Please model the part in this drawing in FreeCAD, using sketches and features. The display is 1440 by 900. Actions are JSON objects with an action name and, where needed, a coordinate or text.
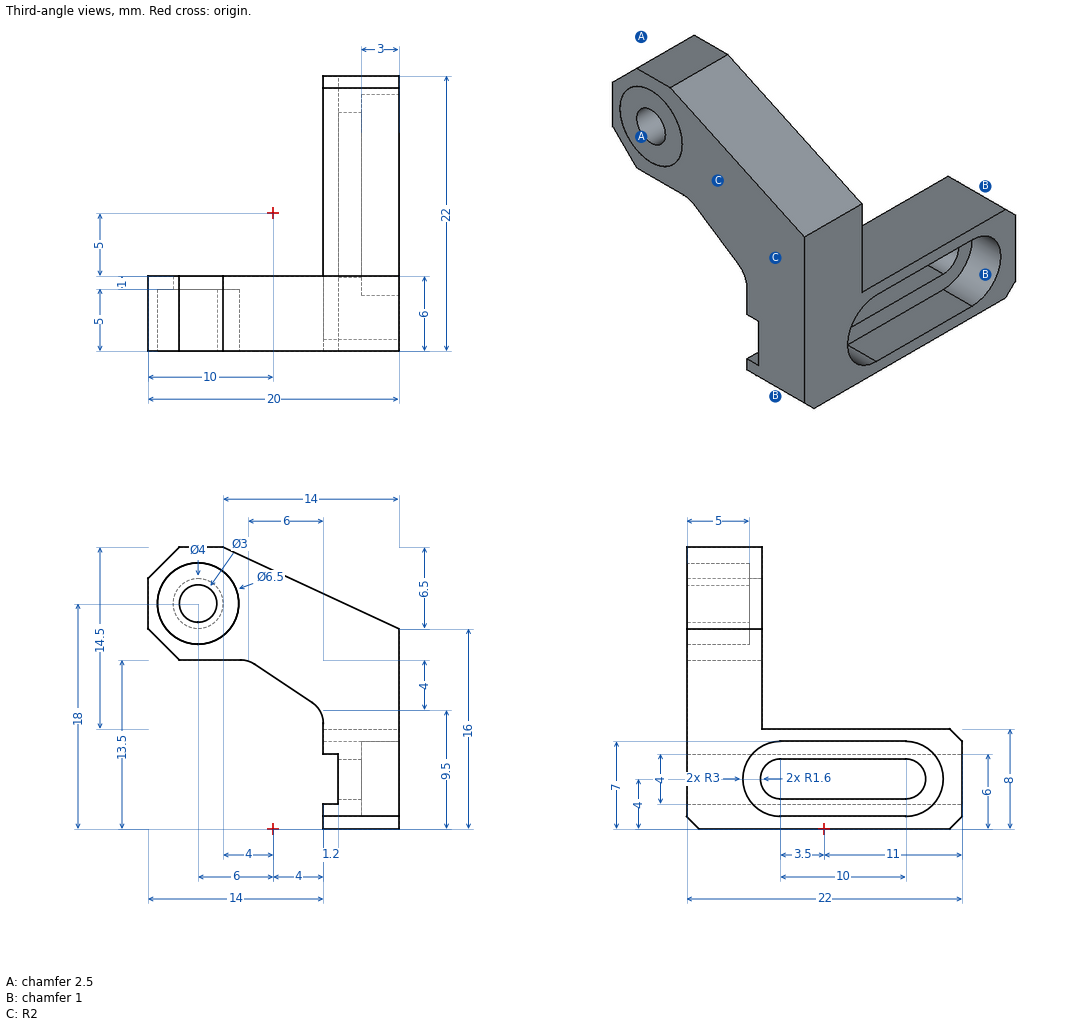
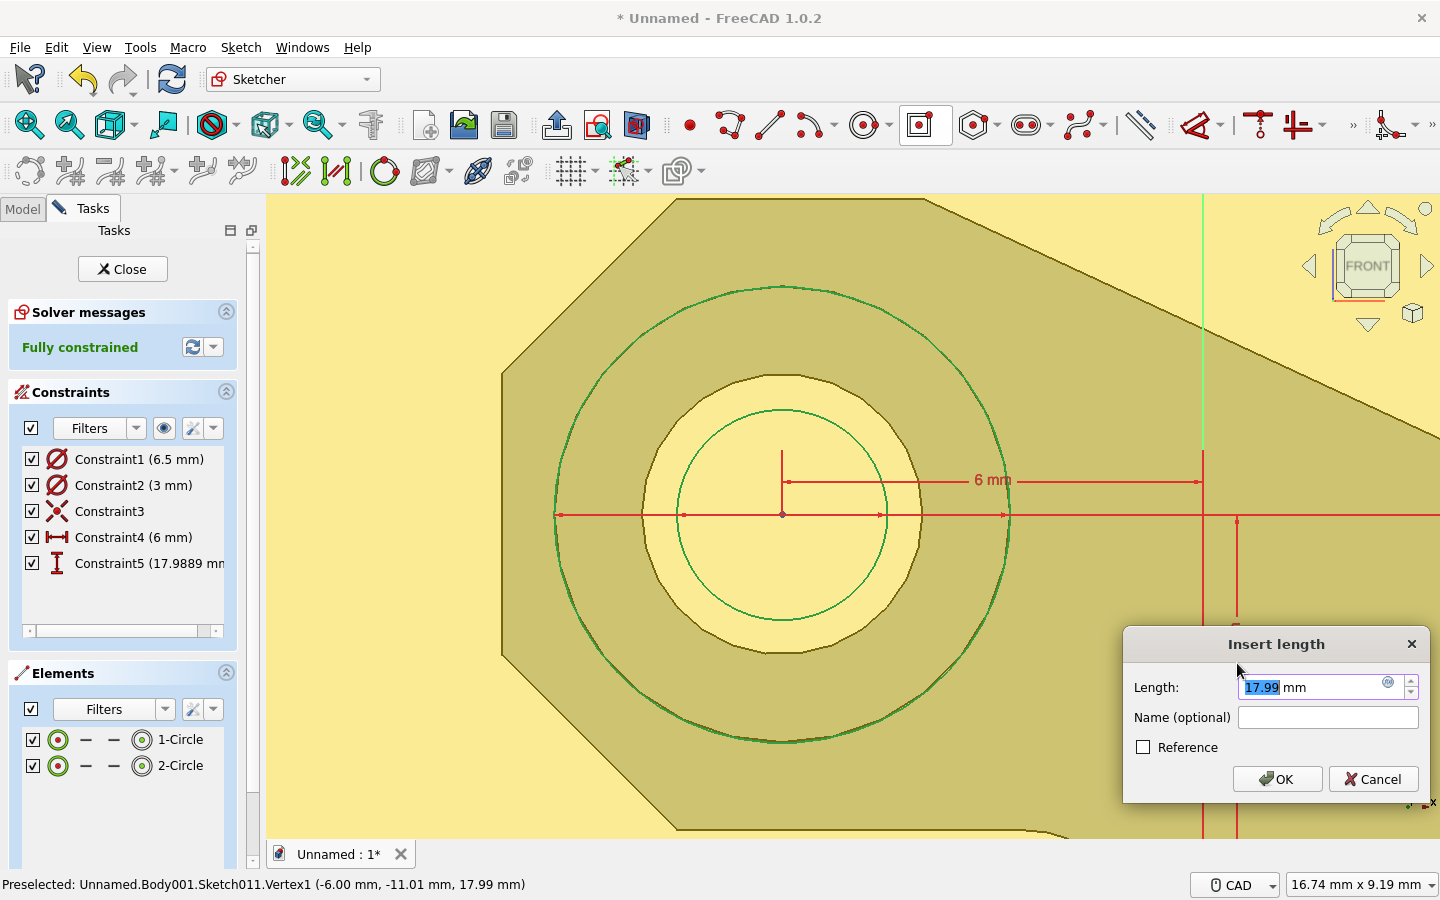
{"action": "type", "text": "18"}
{"action": "key", "text": "Return"}
{"action": "key", "text": "Escape"}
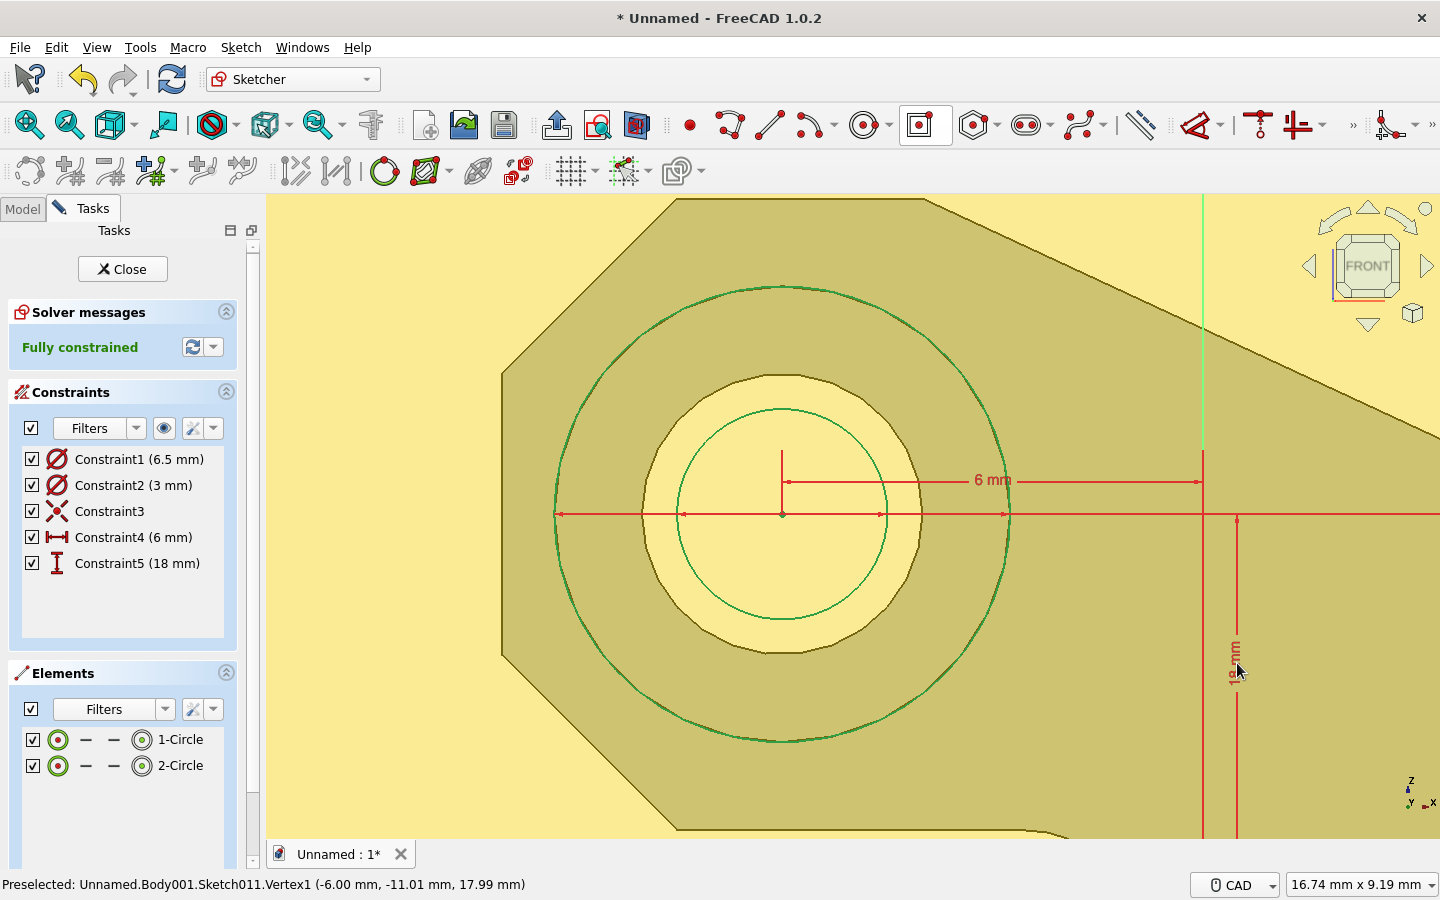
{"action": "left_click", "coordinate": [123, 269]}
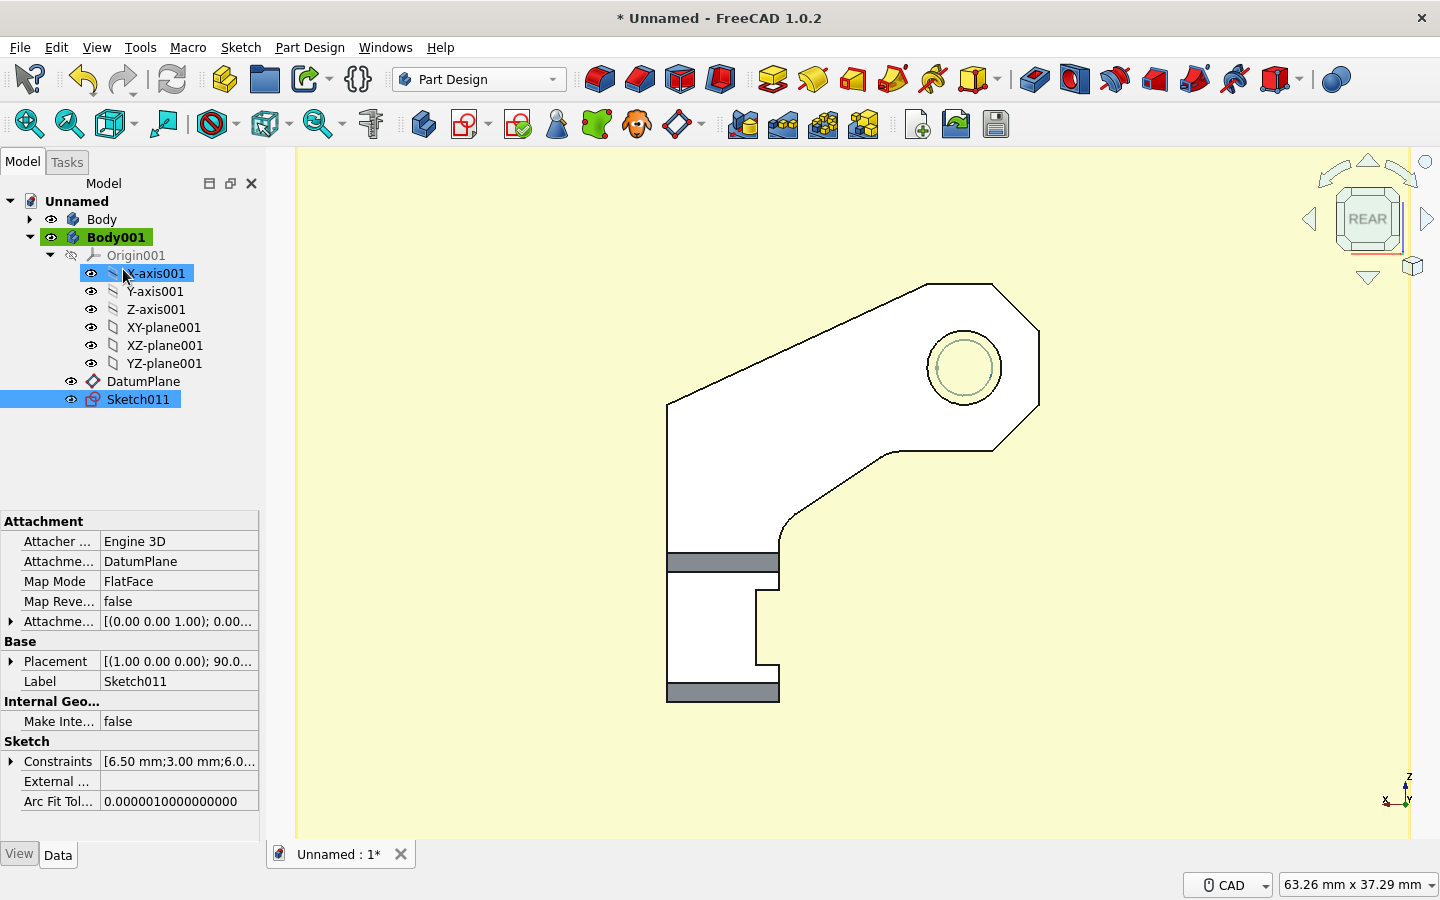
{"action": "left_click", "coordinate": [774, 80]}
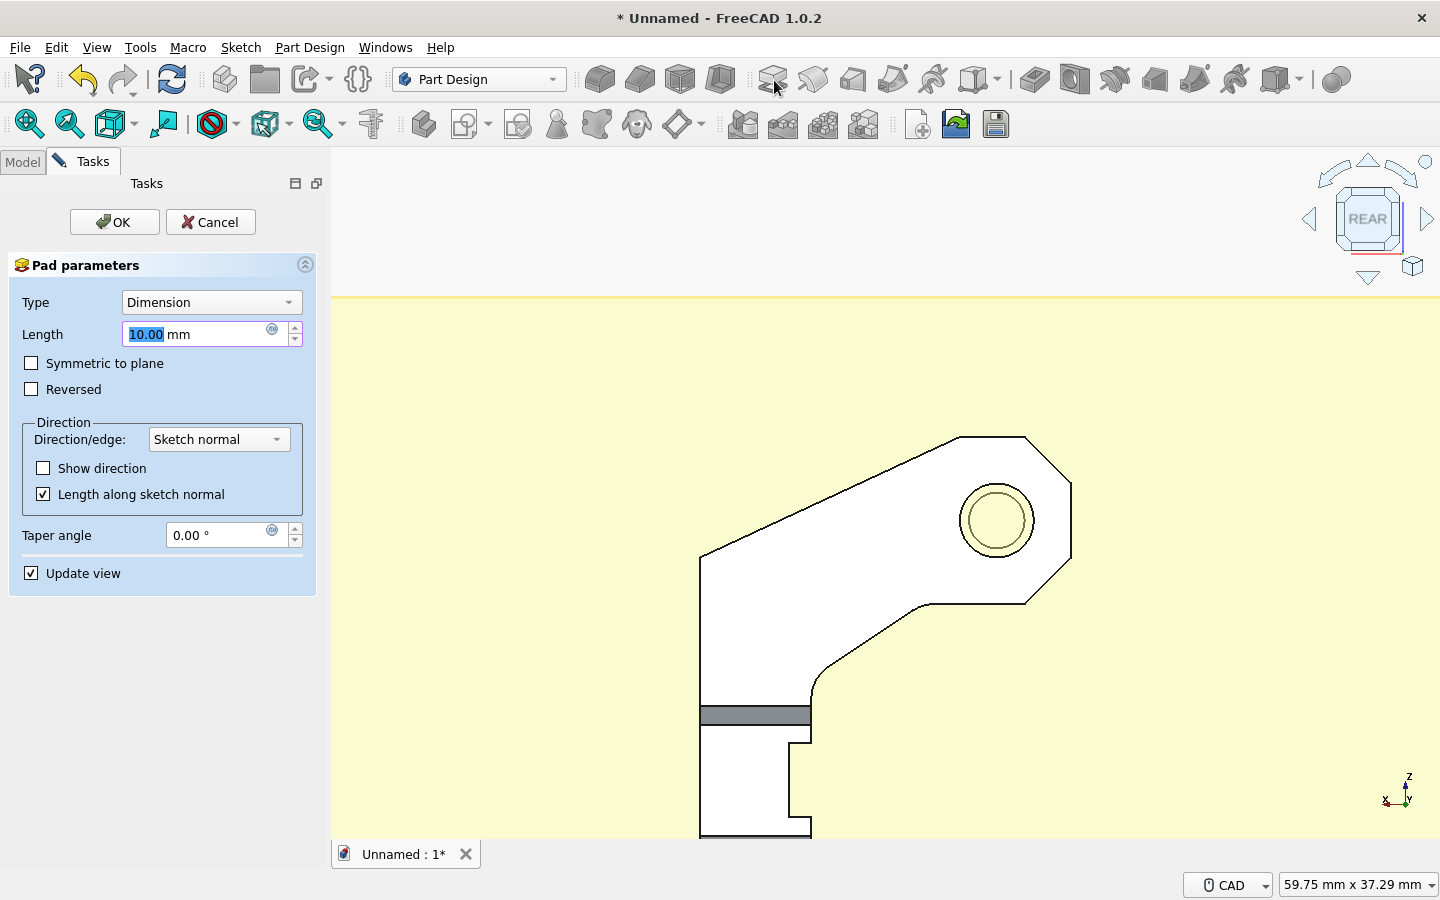
{"action": "type", "text": "5"}
{"action": "key", "text": "Tab"}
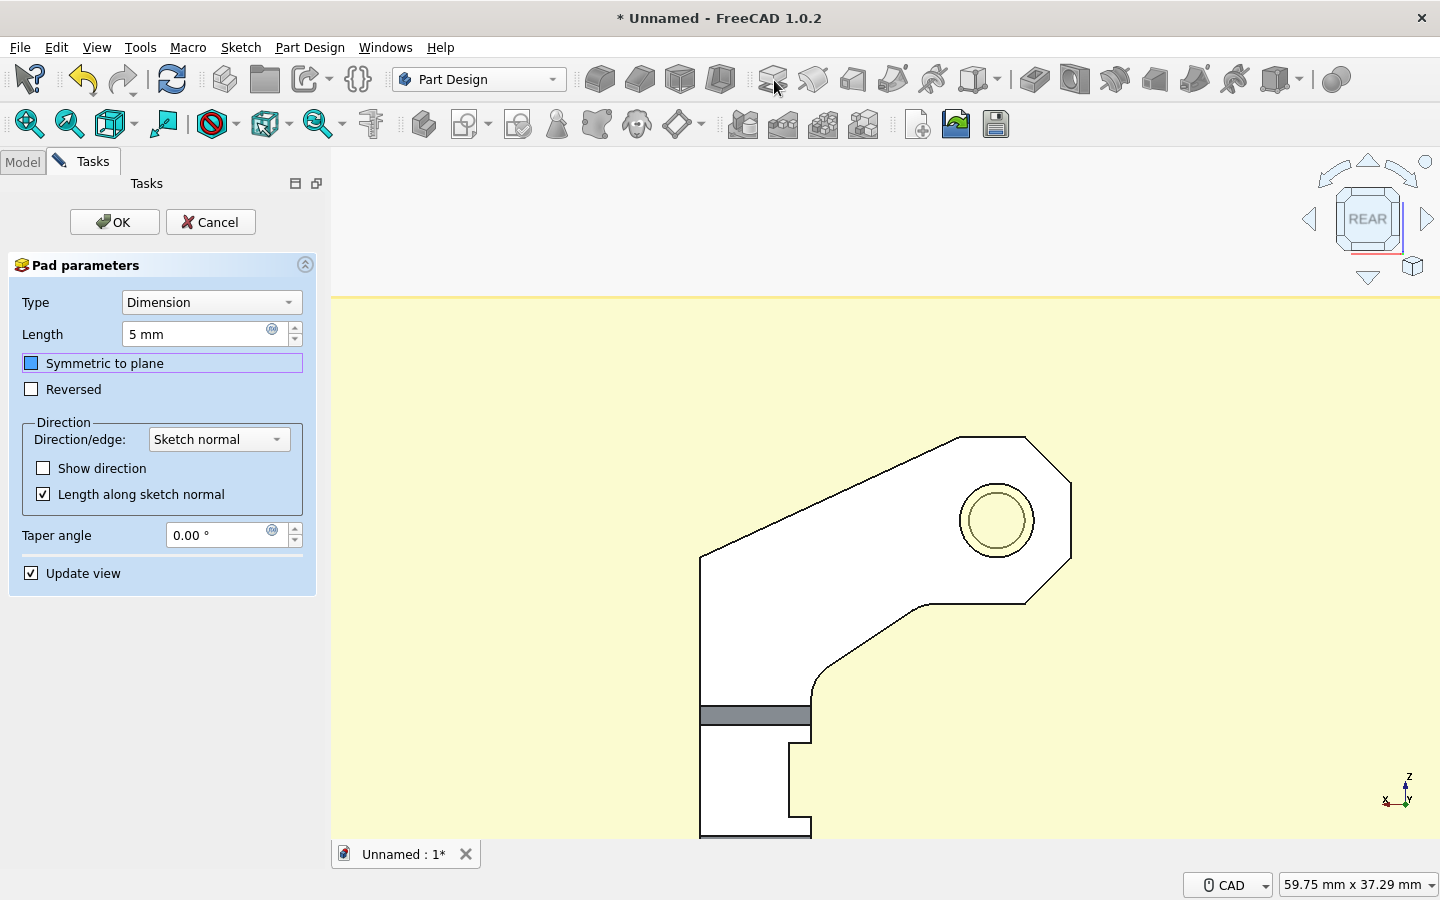
{"action": "left_click", "coordinate": [30, 389]}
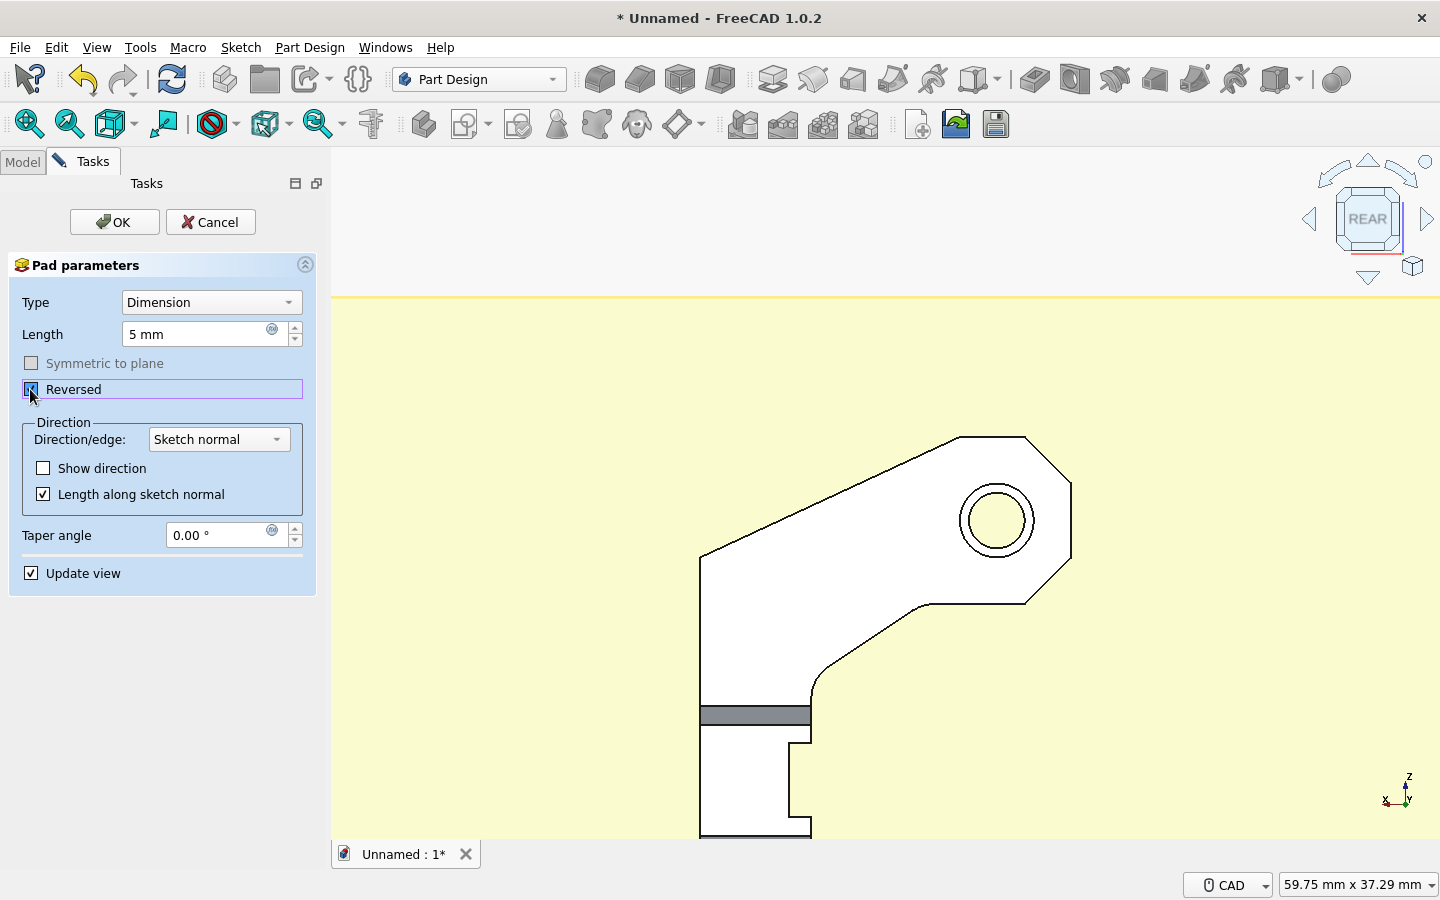
{"action": "left_click", "coordinate": [115, 222]}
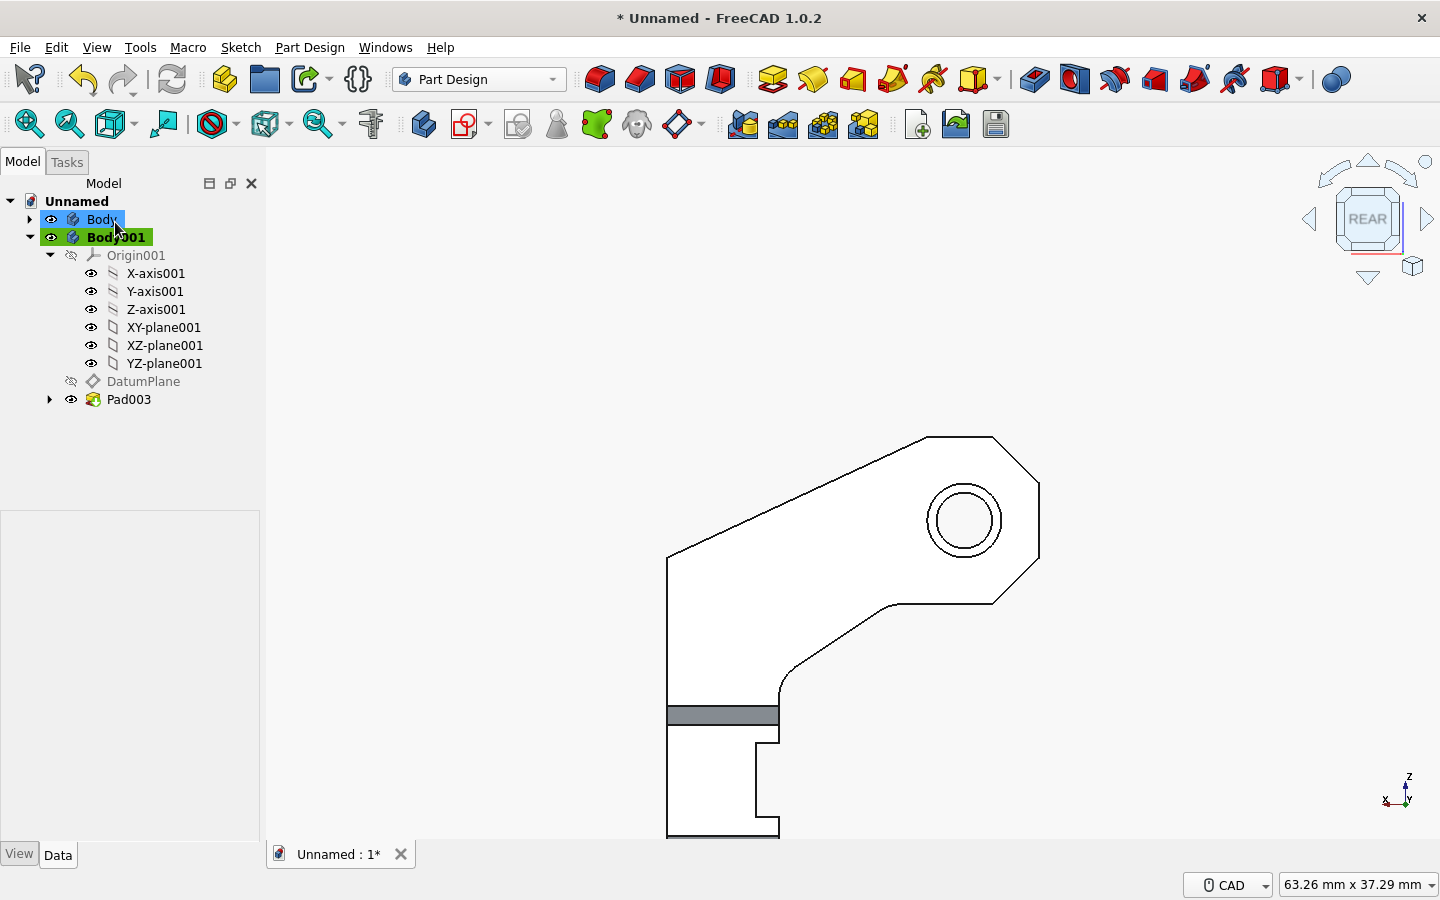
{"action": "key", "text": "0"}